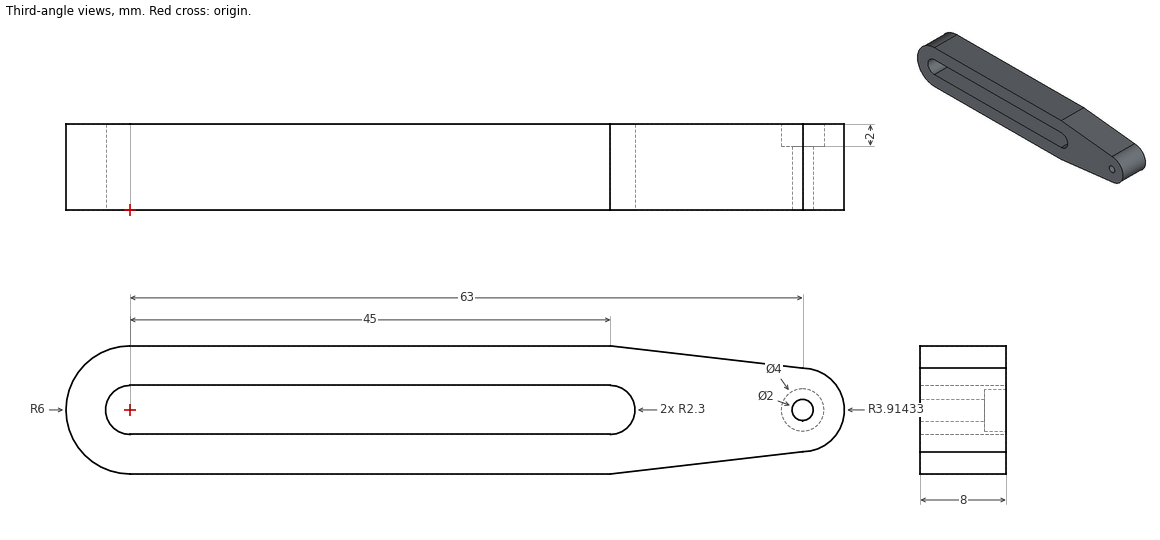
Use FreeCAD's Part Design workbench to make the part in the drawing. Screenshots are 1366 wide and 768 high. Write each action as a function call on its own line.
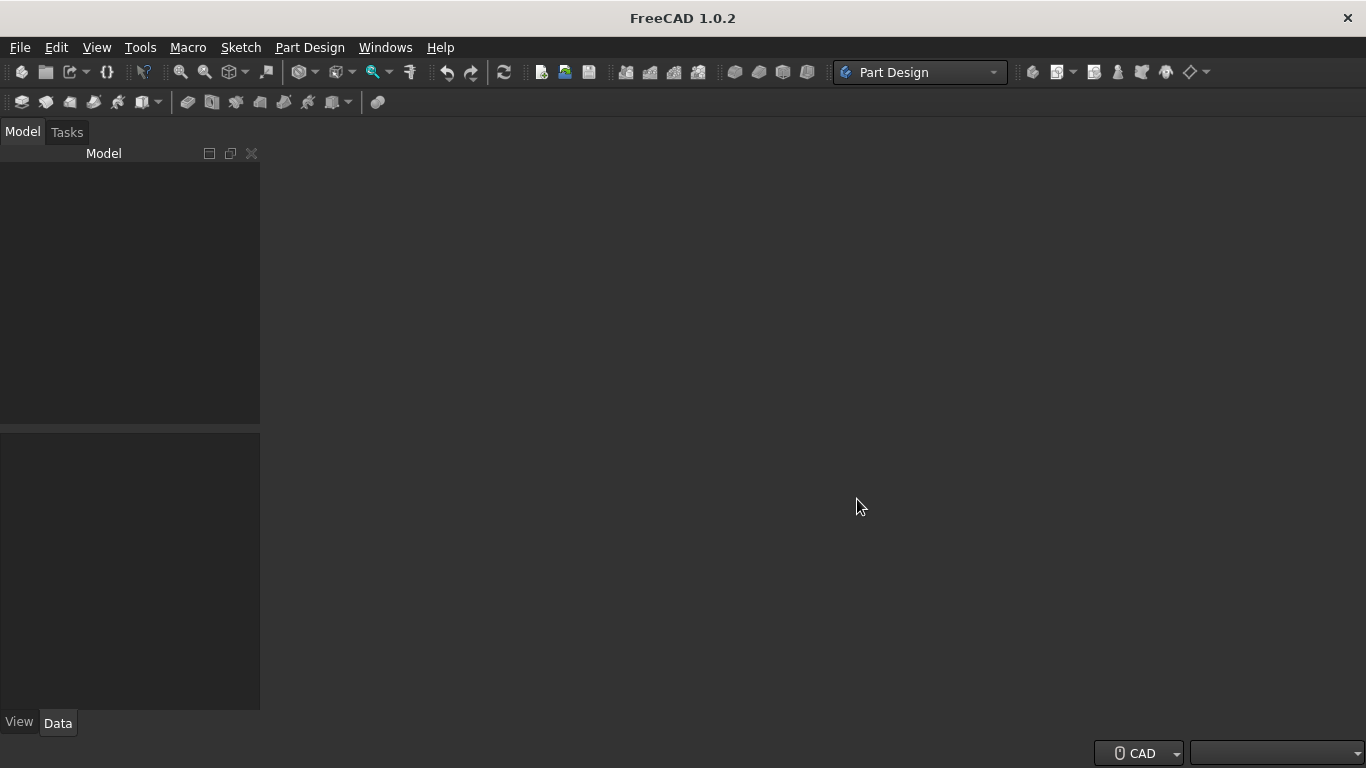
click(542, 72)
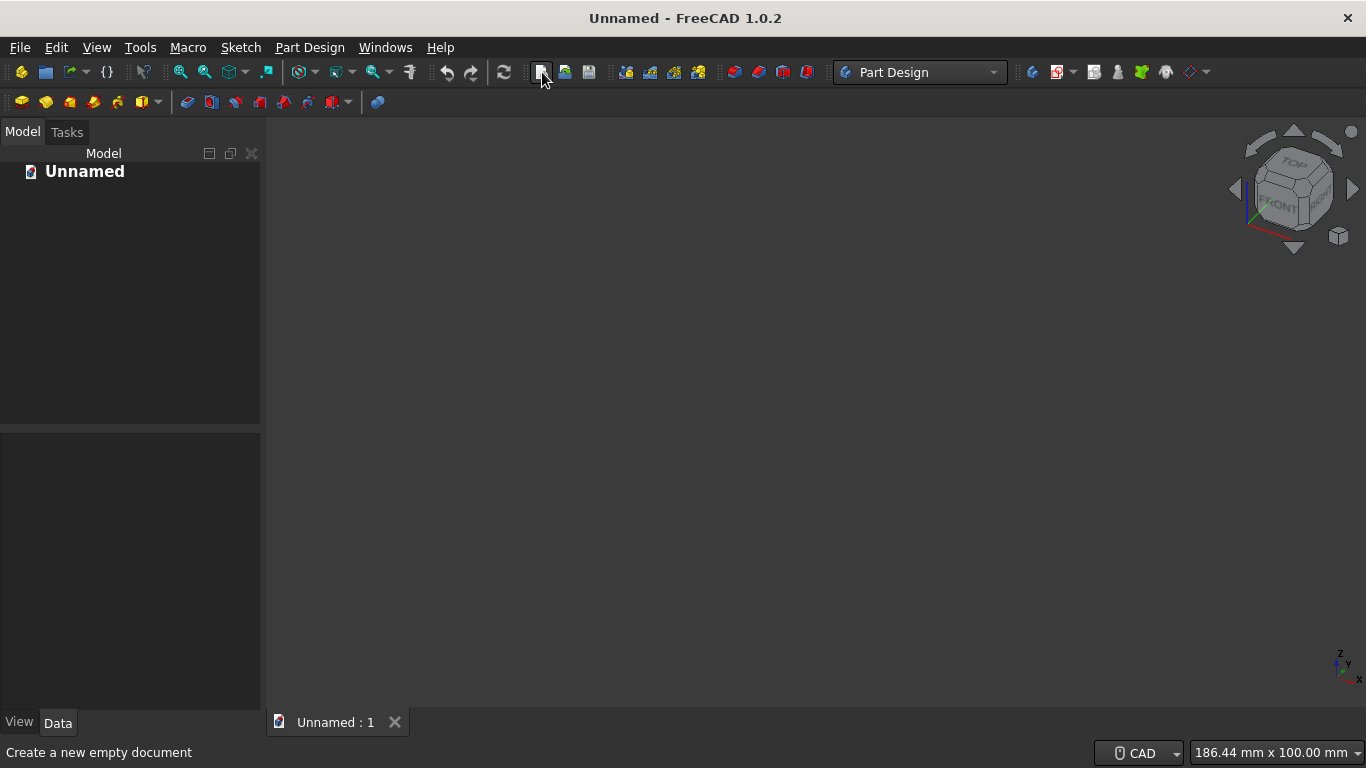
click(1058, 72)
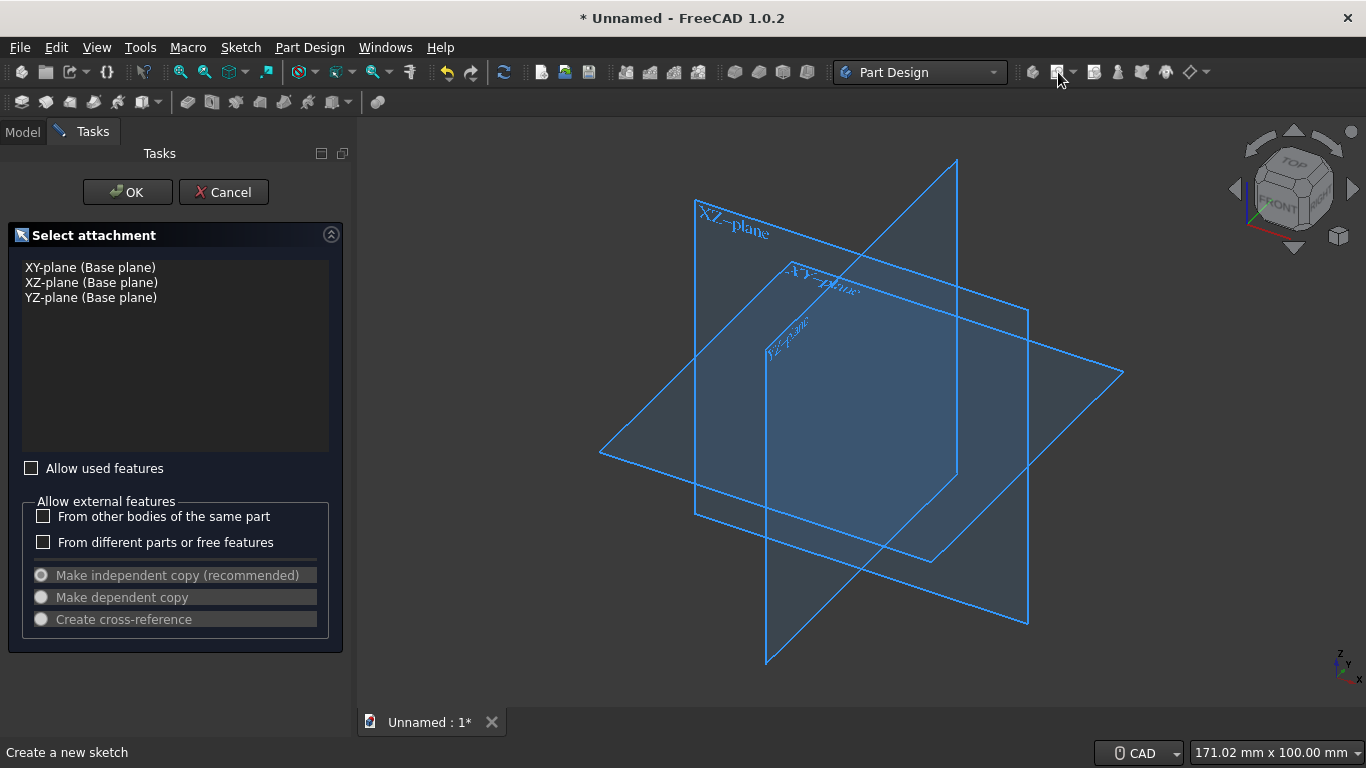
click(82, 282)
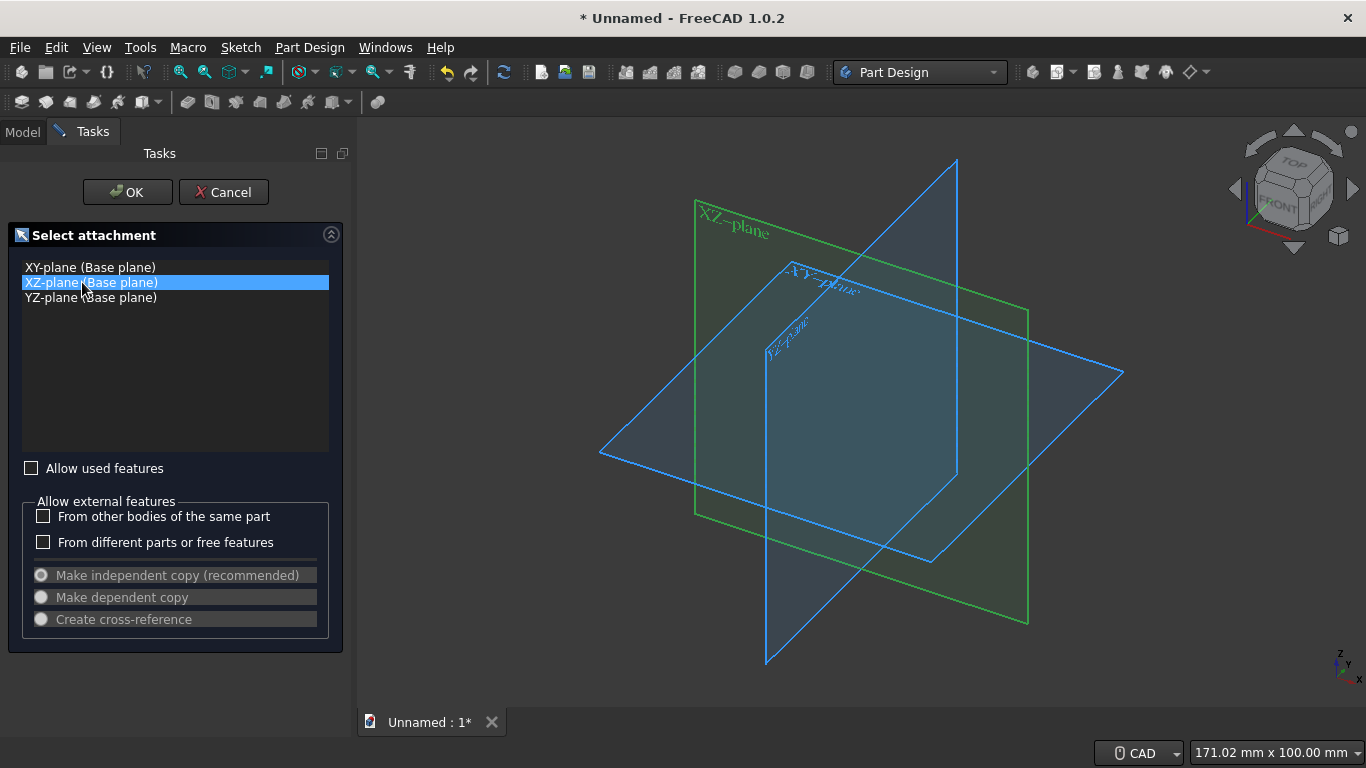
click(128, 192)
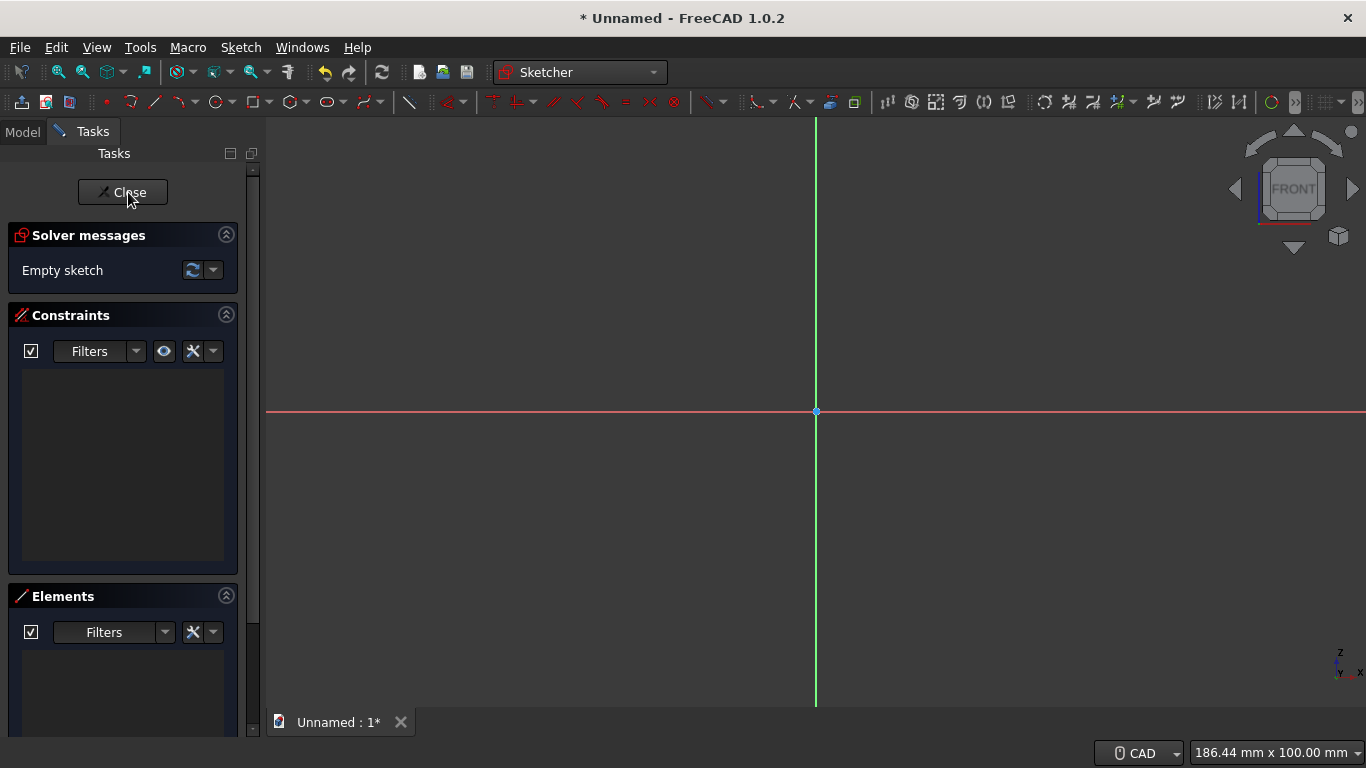
scroll(294, 412, down, 1)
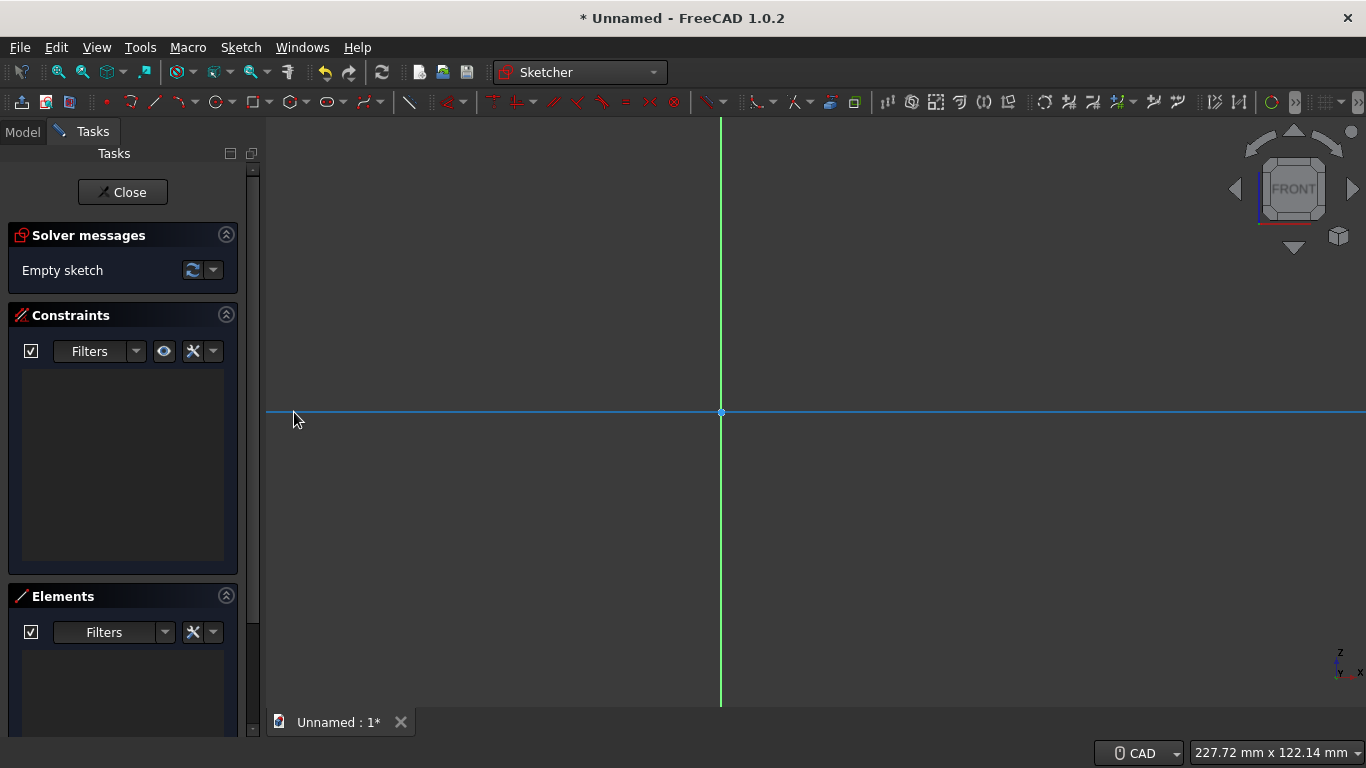
scroll(1016, 412, up, 3)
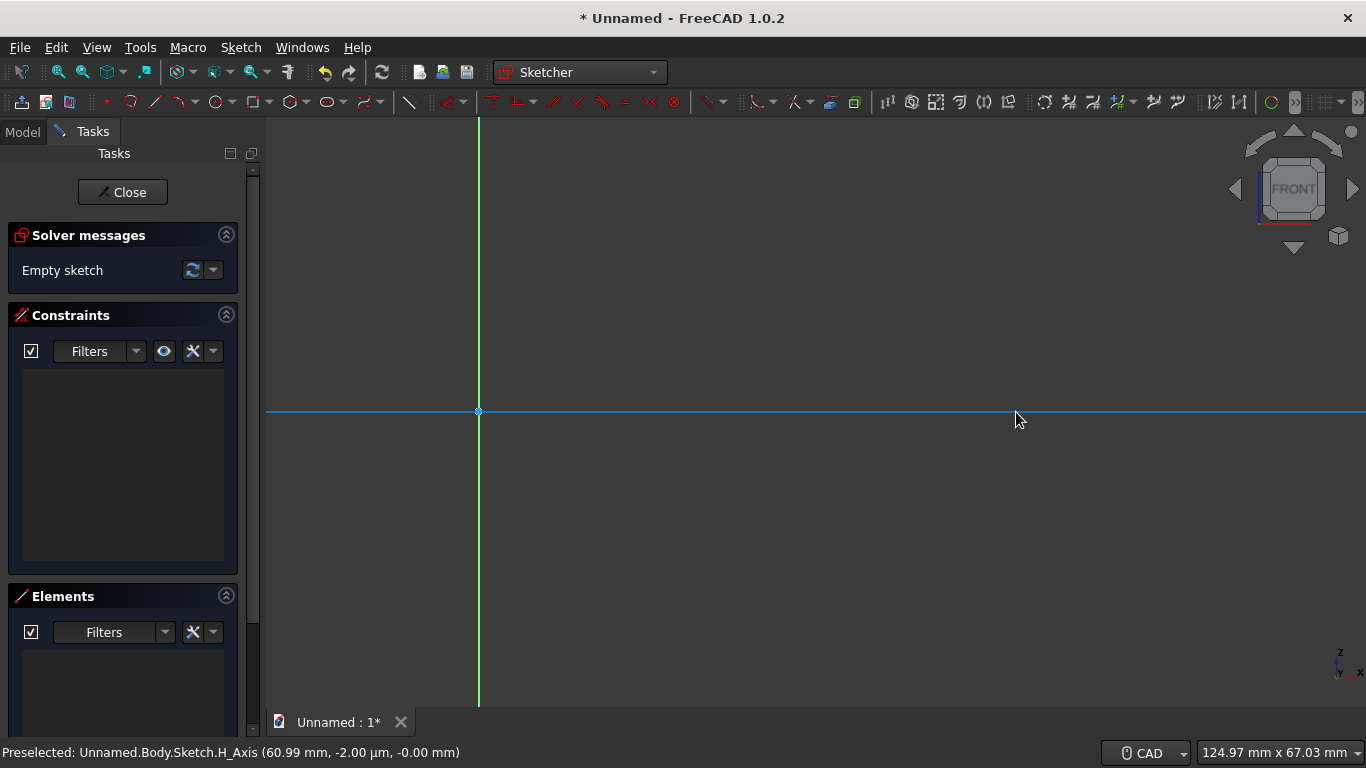
click(132, 102)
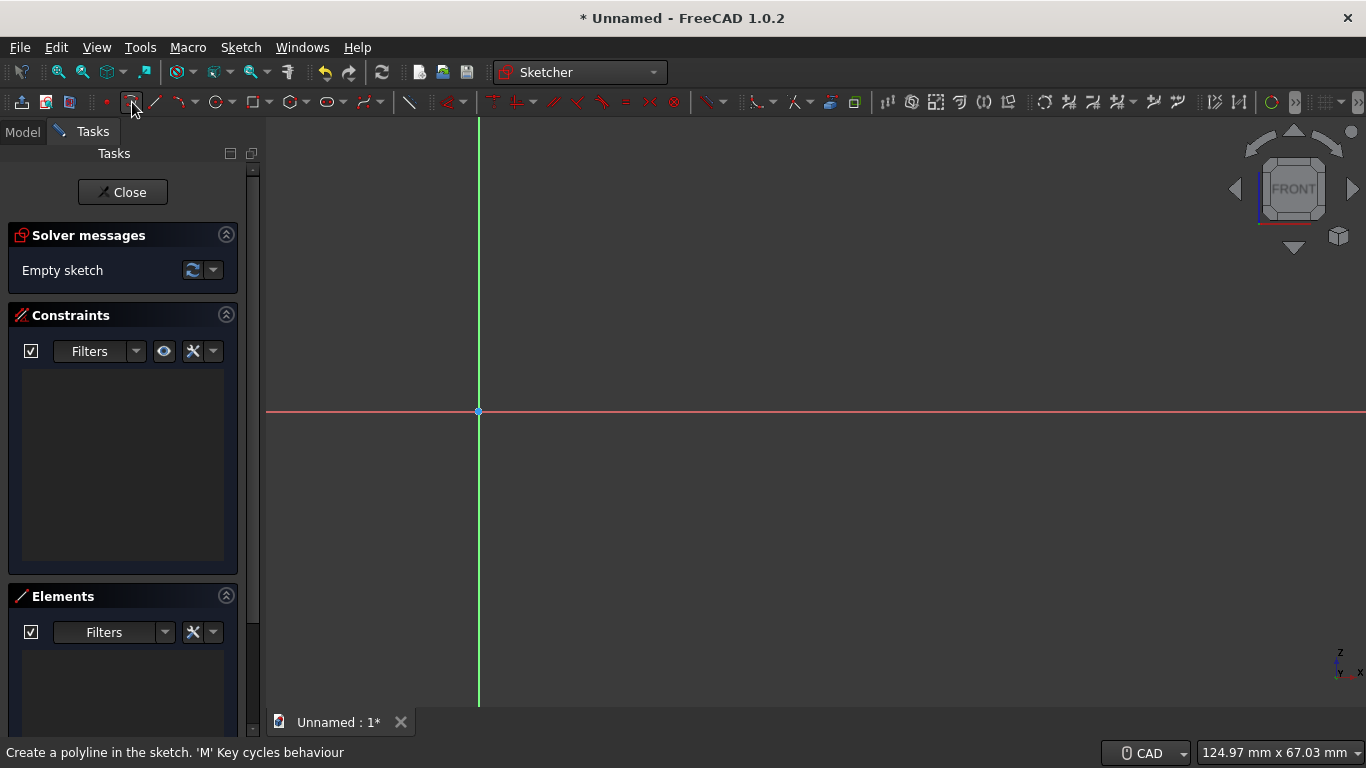
click(479, 359)
click(875, 359)
click(1033, 377)
right_click(1033, 377)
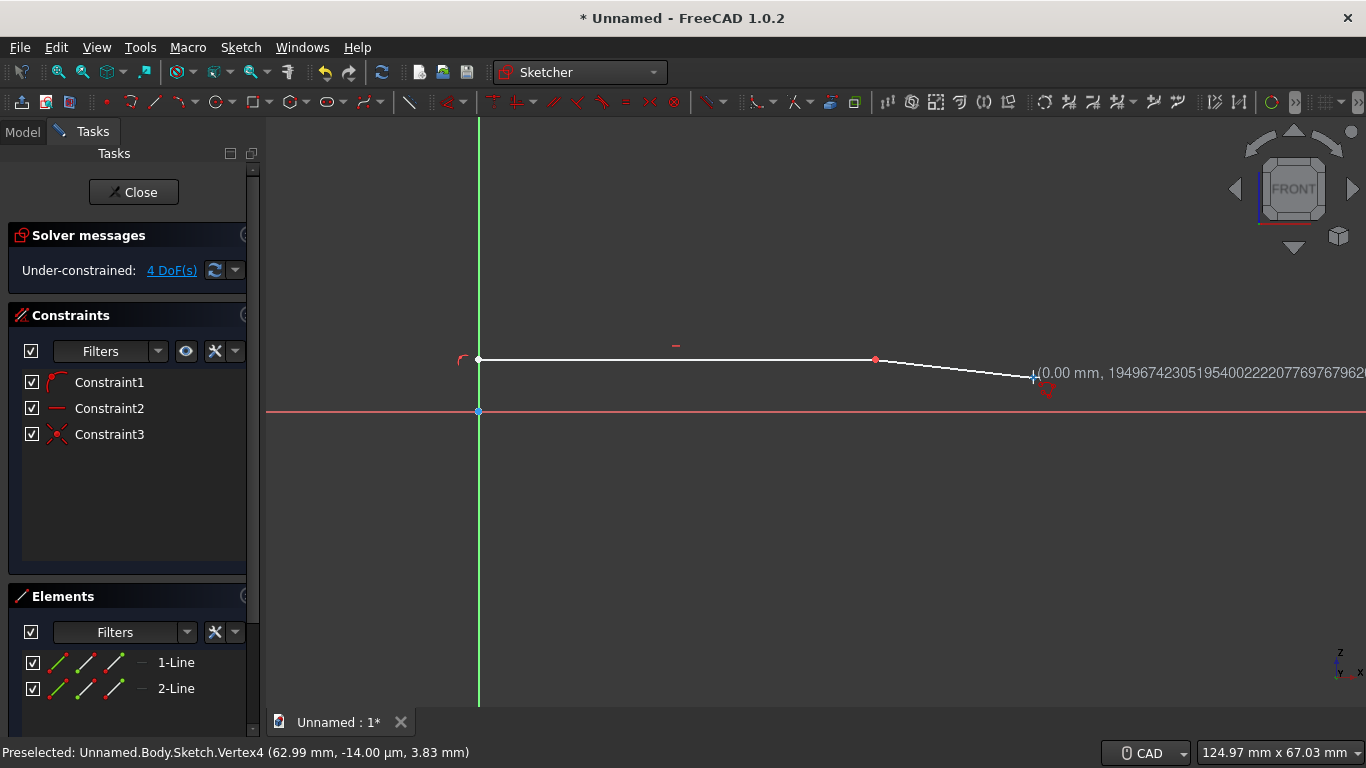
click(1033, 446)
click(875, 465)
click(479, 465)
right_click(479, 465)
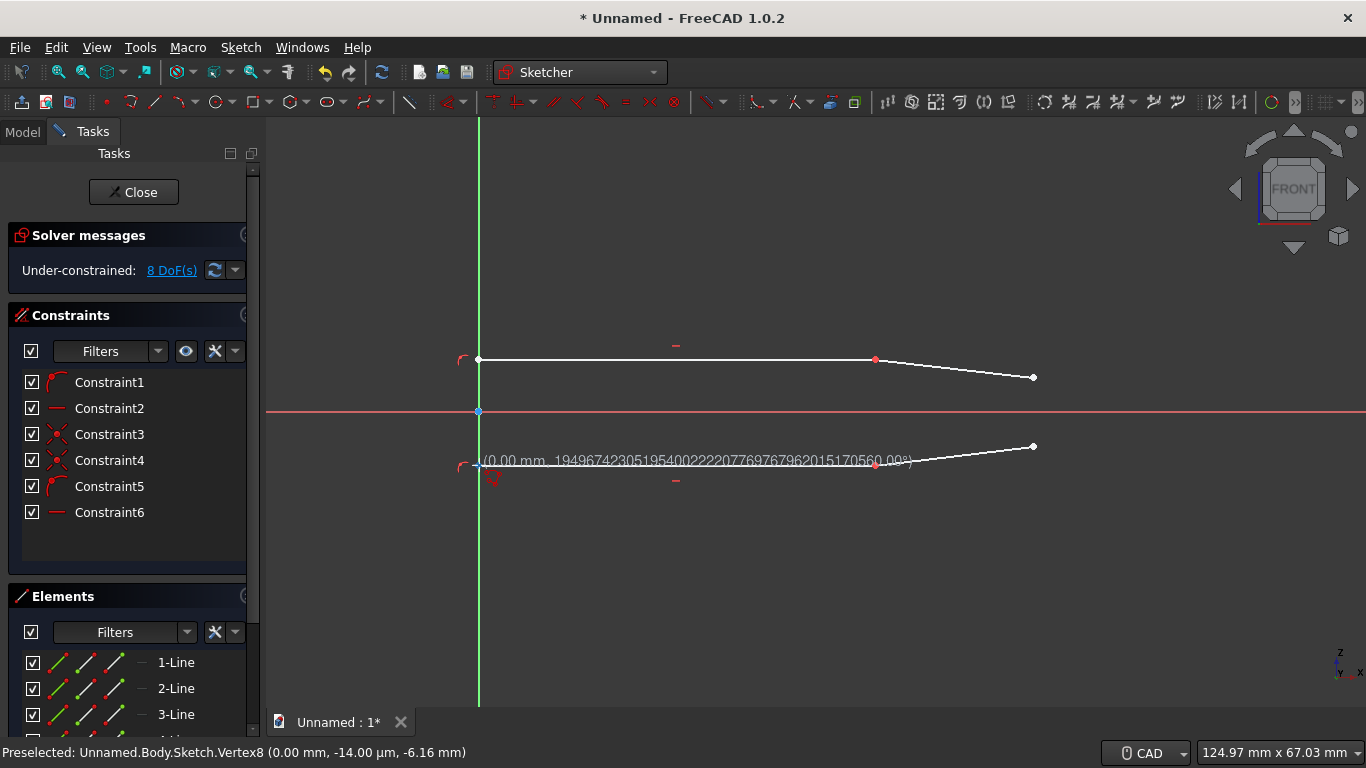
click(180, 102)